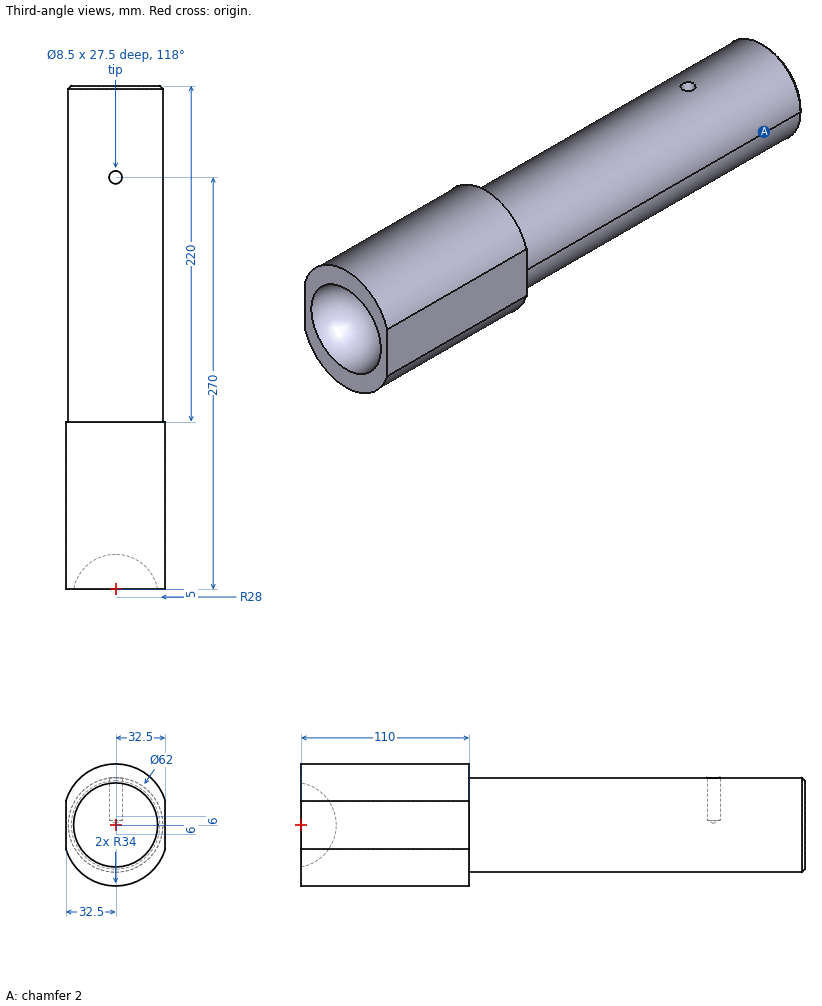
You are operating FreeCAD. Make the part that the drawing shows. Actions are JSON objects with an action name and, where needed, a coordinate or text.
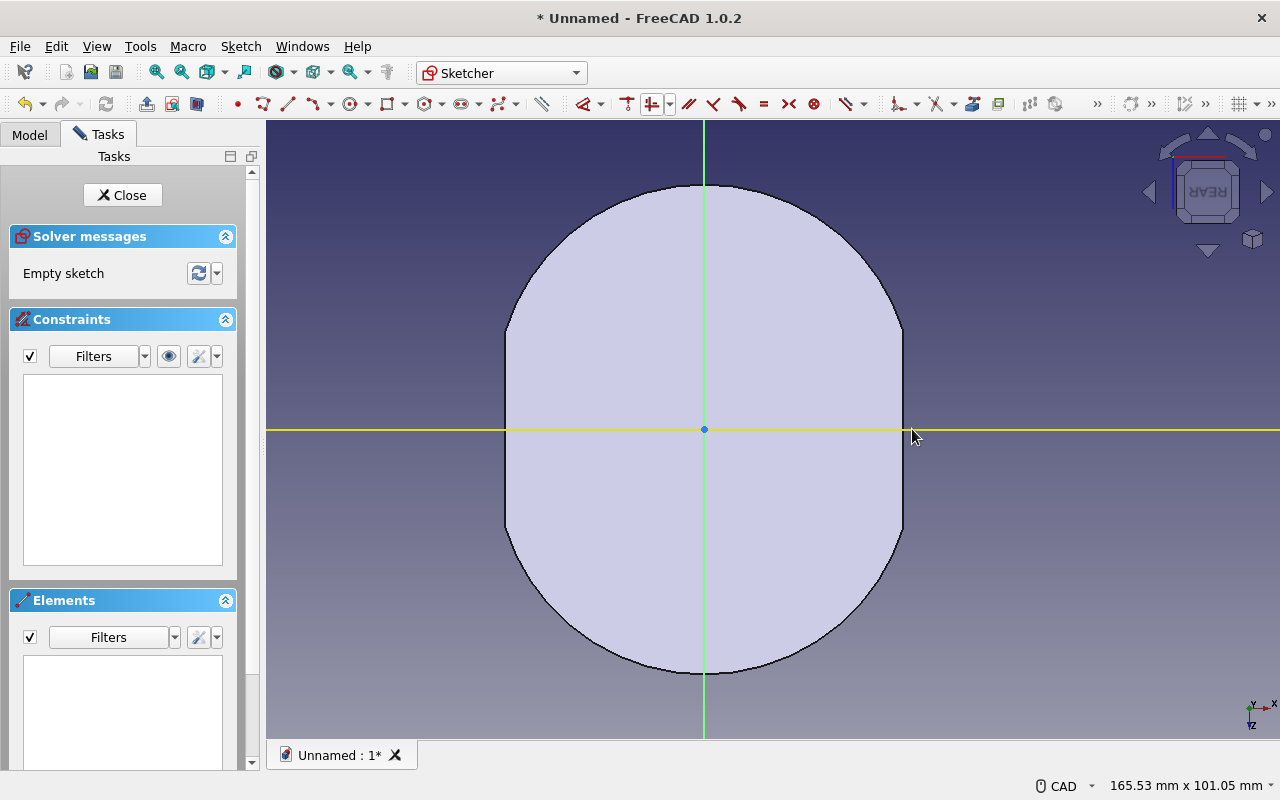
{"action": "left_click", "coordinate": [350, 104]}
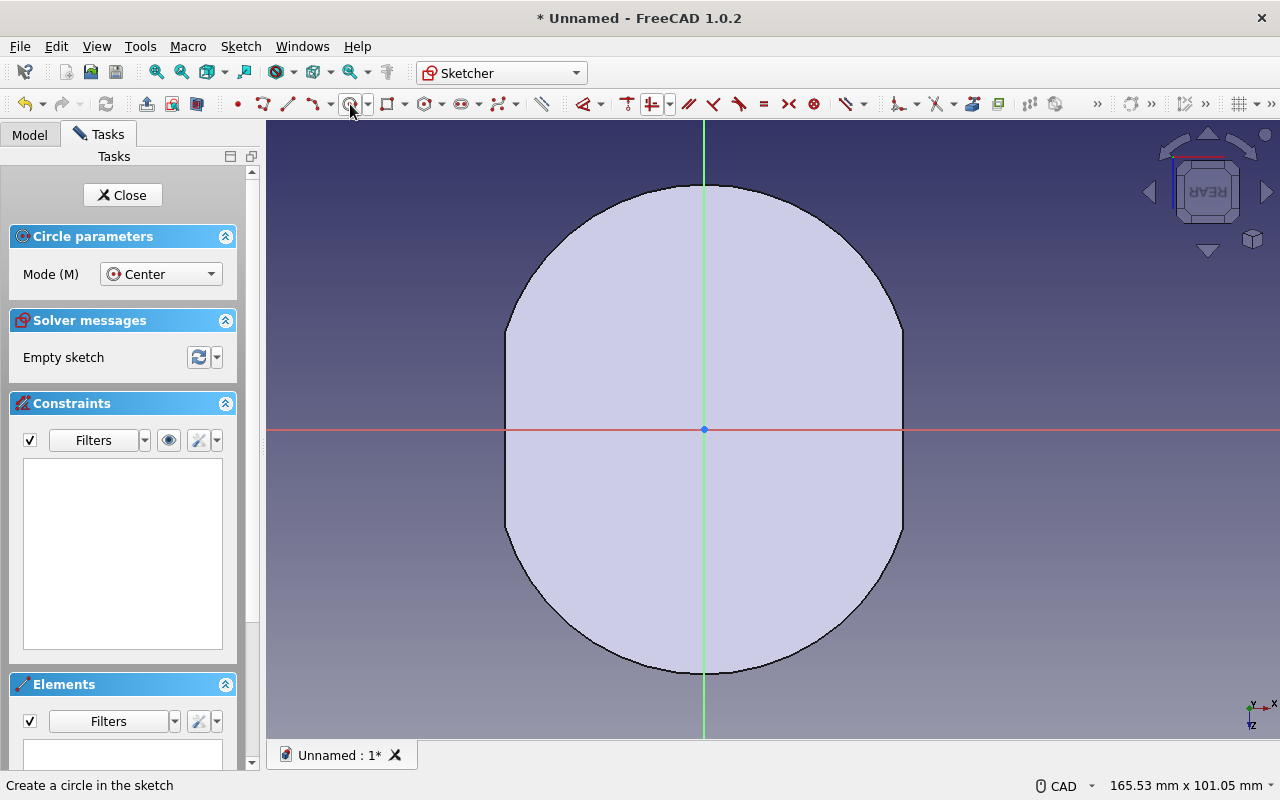
{"action": "left_click", "coordinate": [704, 429]}
{"action": "mouse_move", "coordinate": [839, 295]}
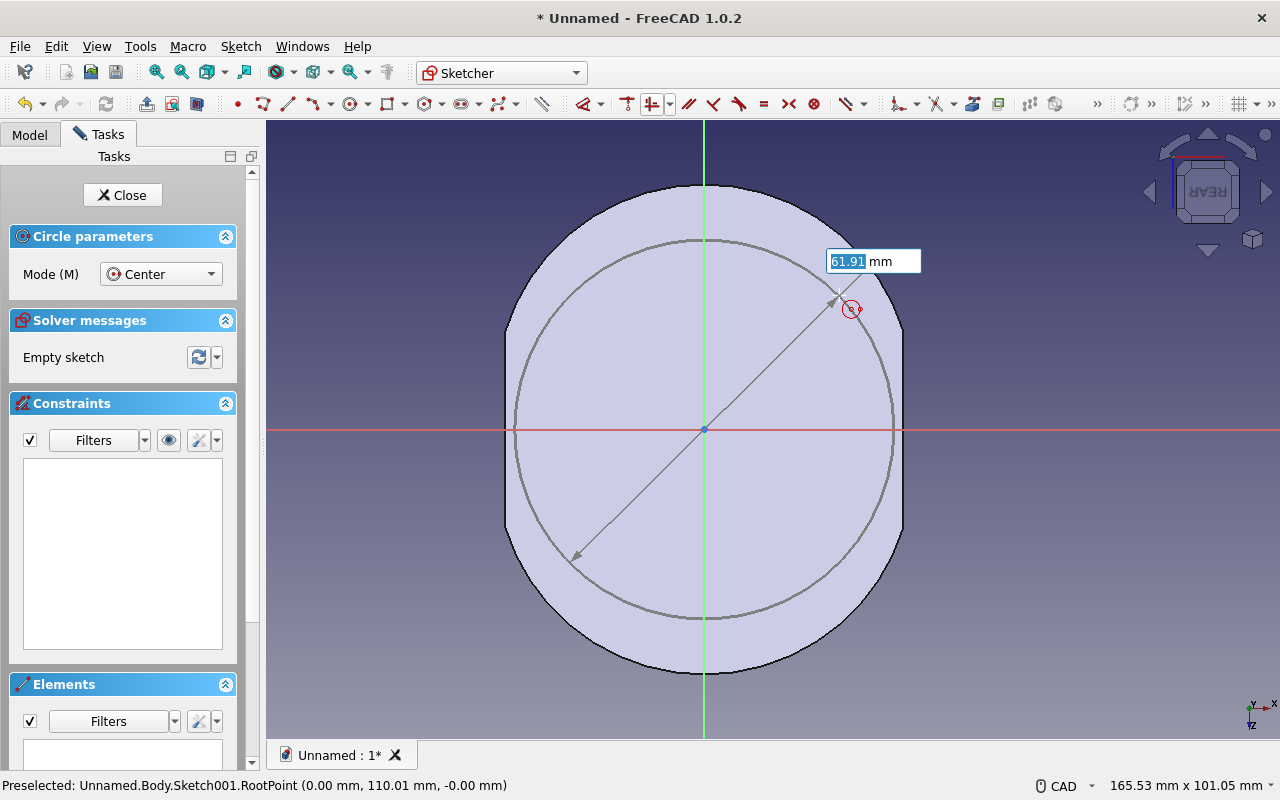
{"action": "type", "text": "62"}
{"action": "key", "text": "Return"}
{"action": "key", "text": "Escape"}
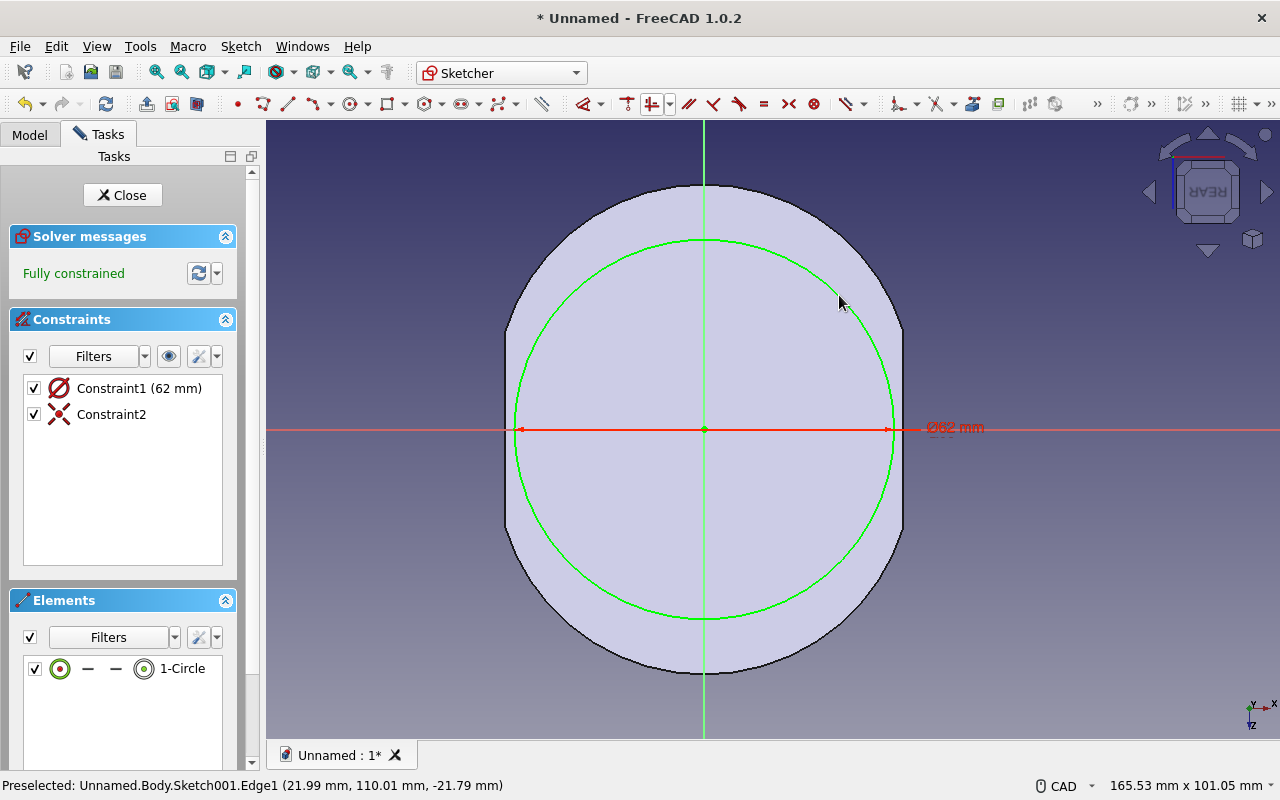
{"action": "left_click", "coordinate": [123, 195]}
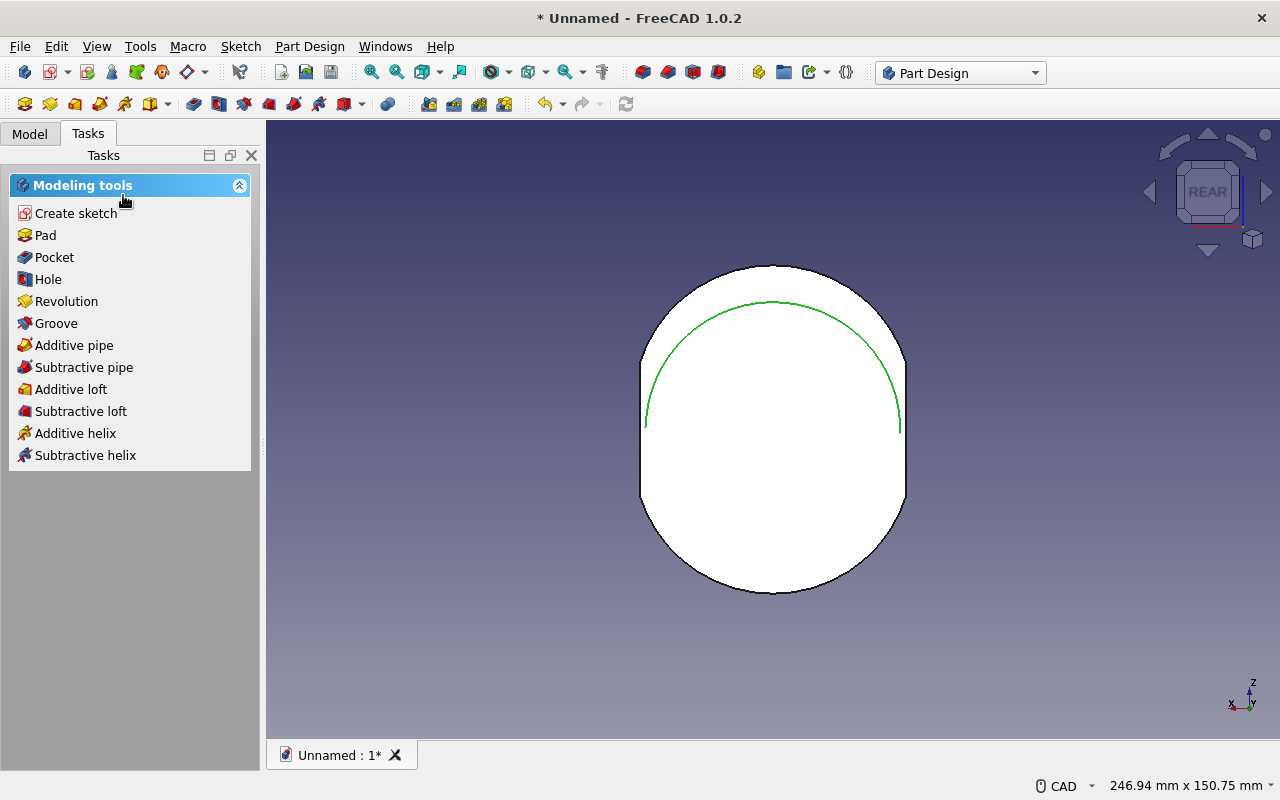
{"action": "left_click", "coordinate": [25, 104]}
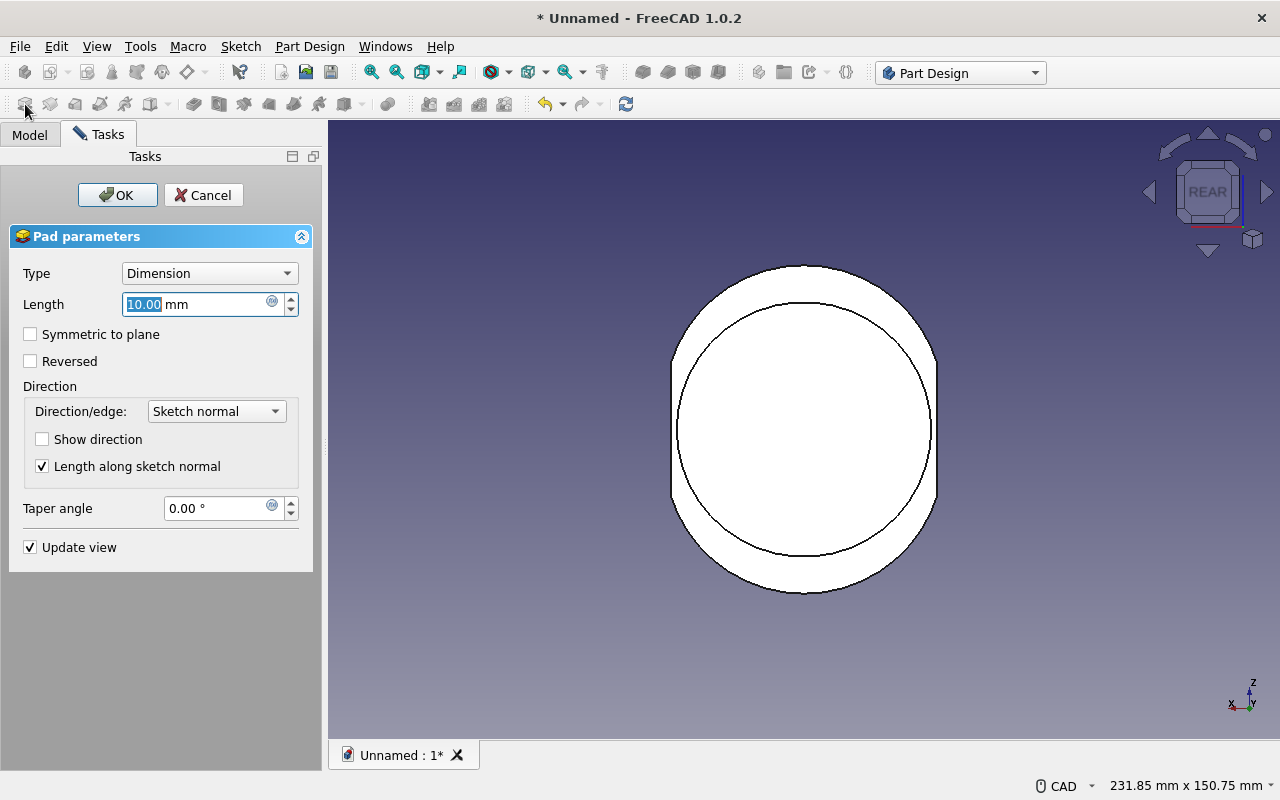
{"action": "type", "text": "220"}
{"action": "key", "text": "Tab"}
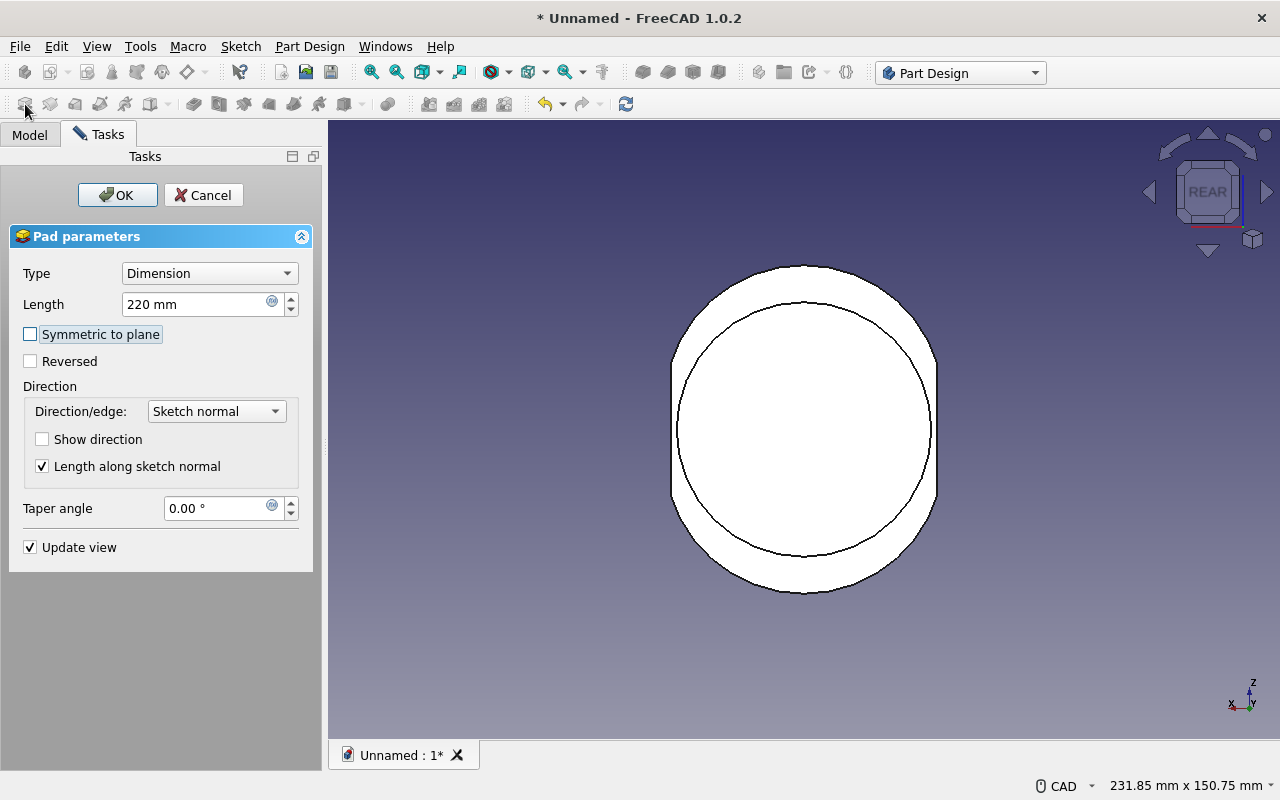
{"action": "left_click", "coordinate": [118, 195]}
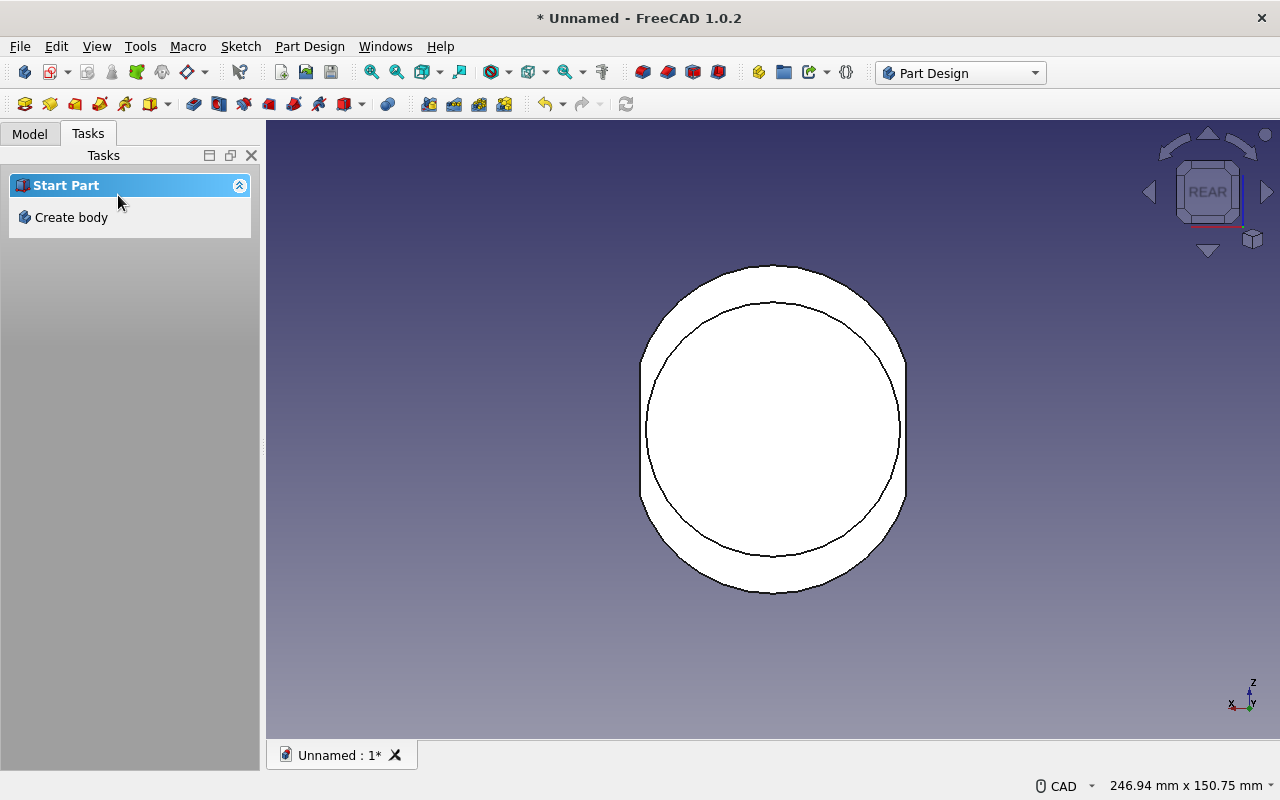
{"action": "left_click", "coordinate": [30, 134]}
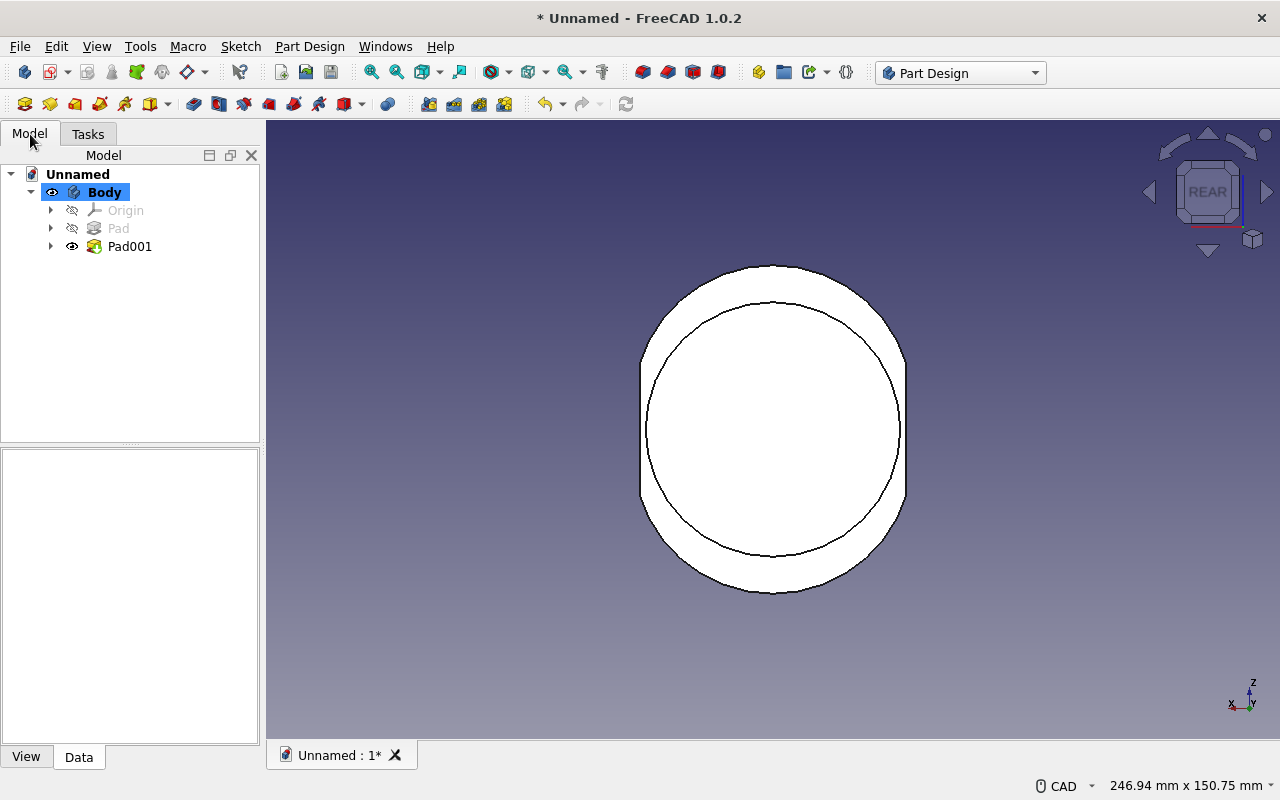
{"action": "left_click", "coordinate": [51, 210]}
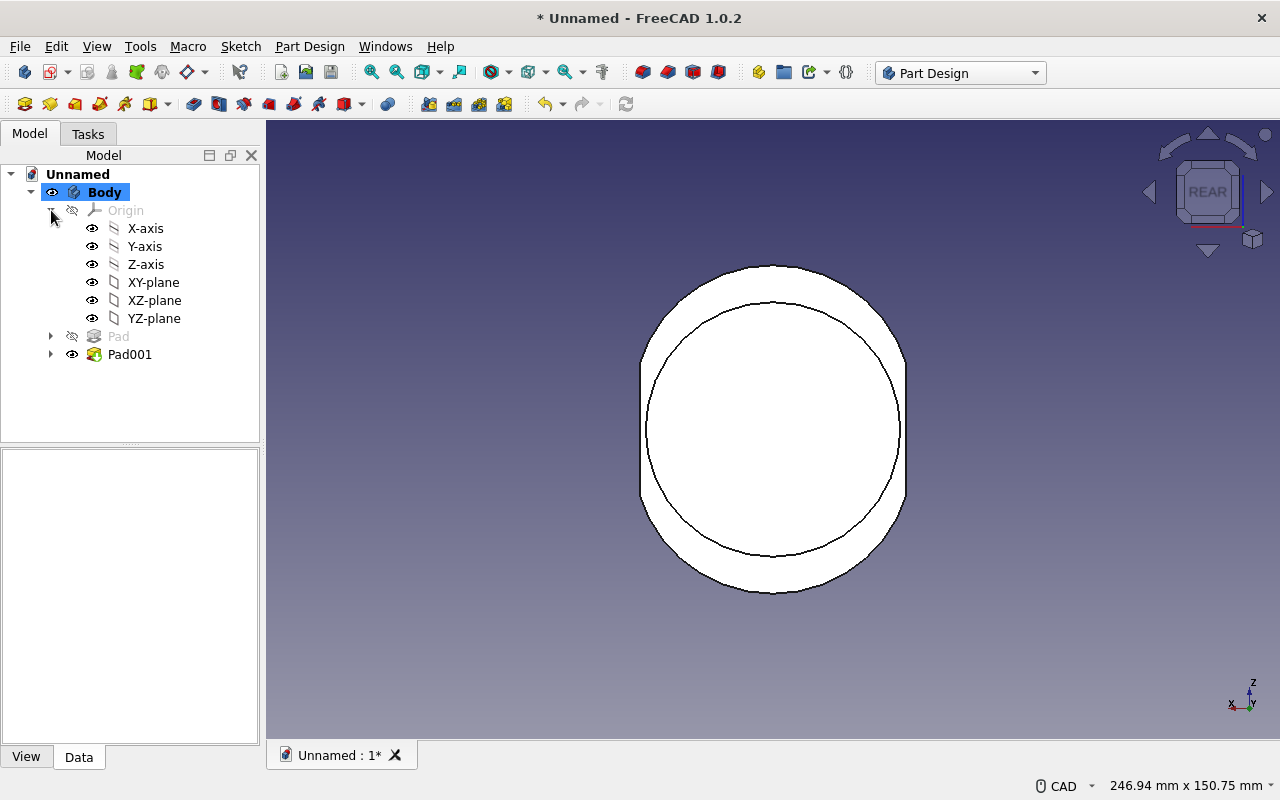
{"action": "left_click", "coordinate": [137, 282]}